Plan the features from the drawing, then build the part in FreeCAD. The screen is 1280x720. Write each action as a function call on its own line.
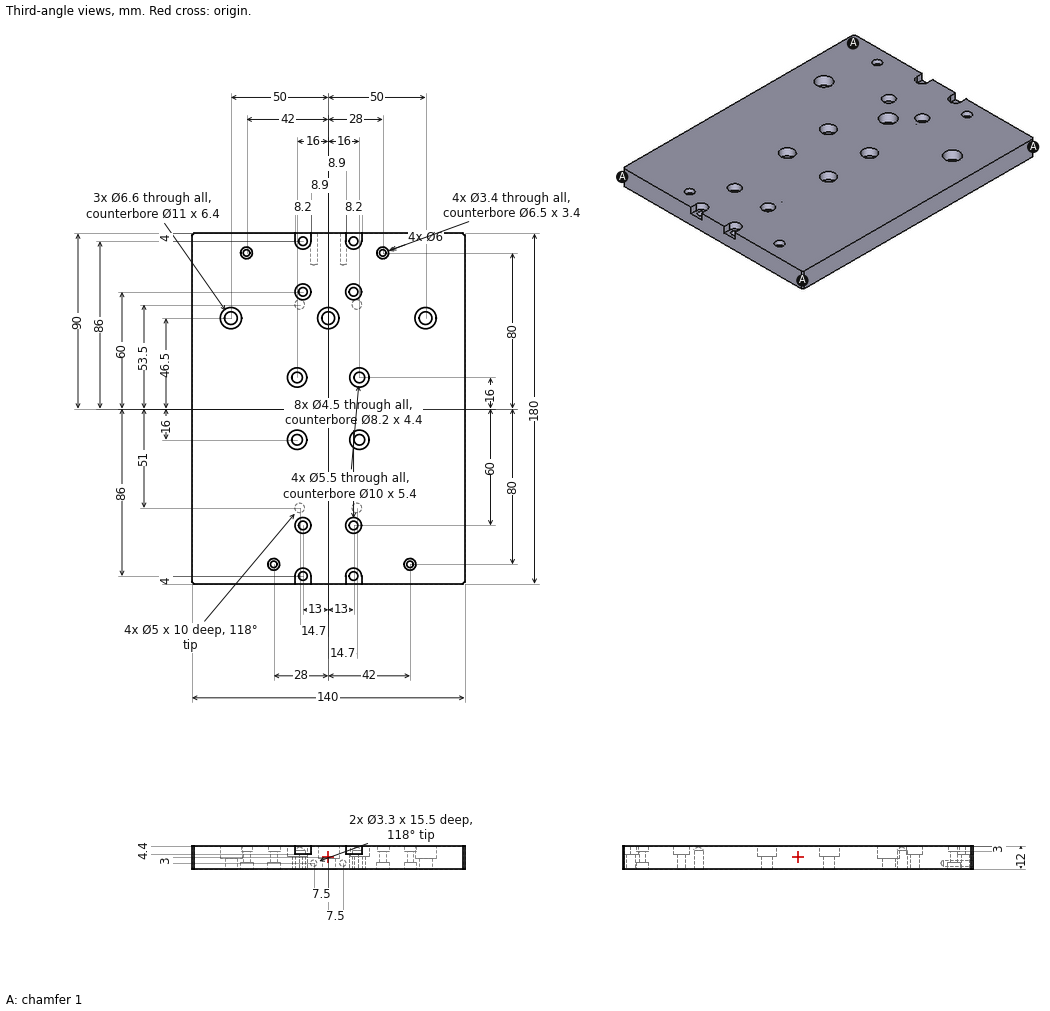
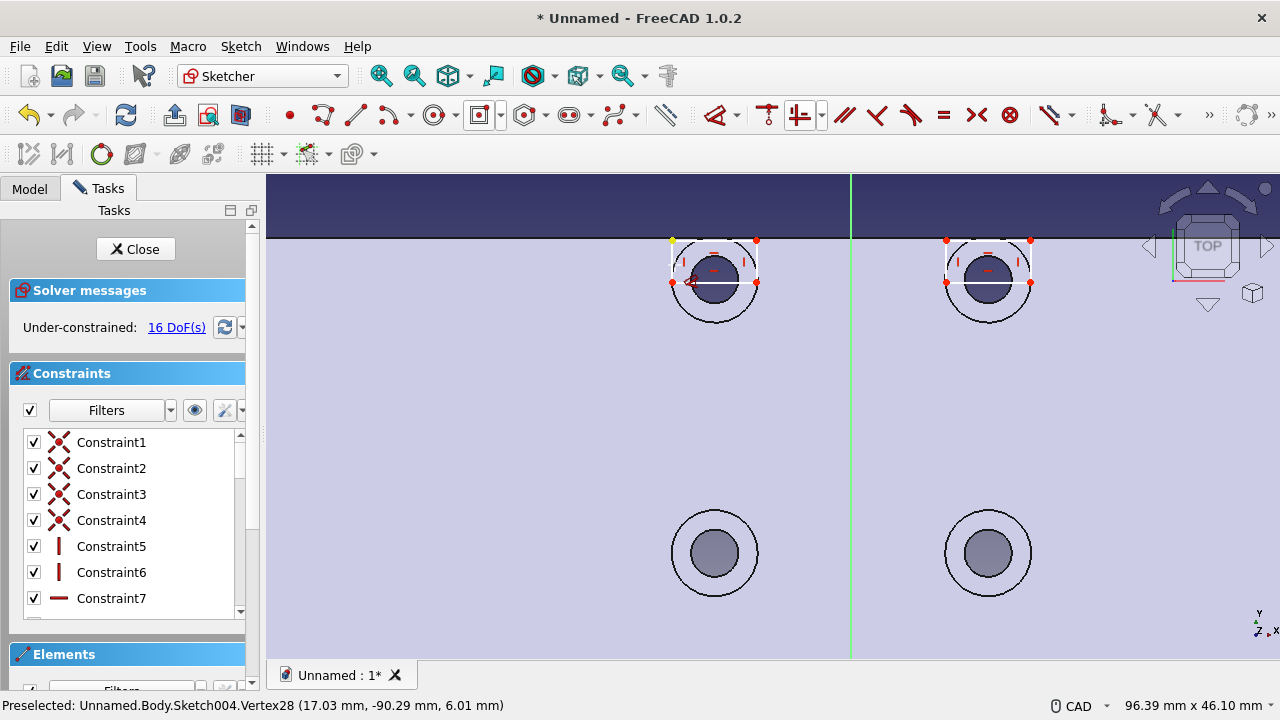
click(672, 262)
click(638, 262)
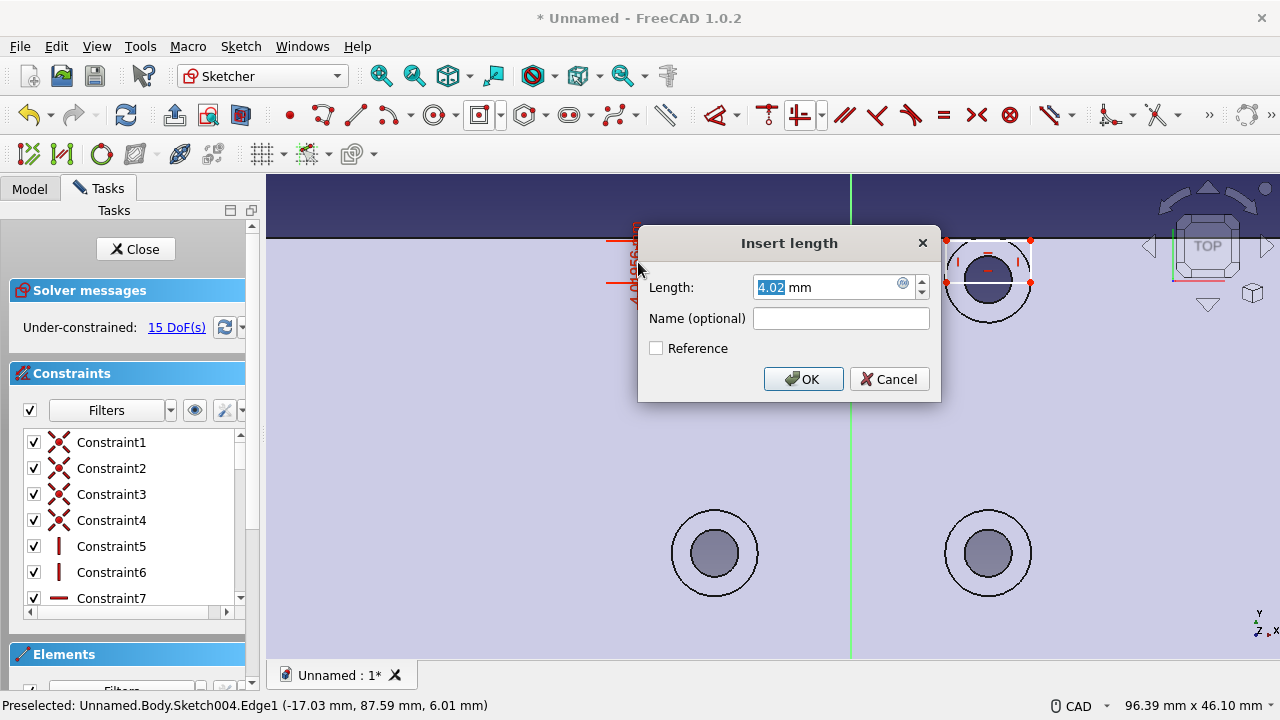
text(4)
key(Return)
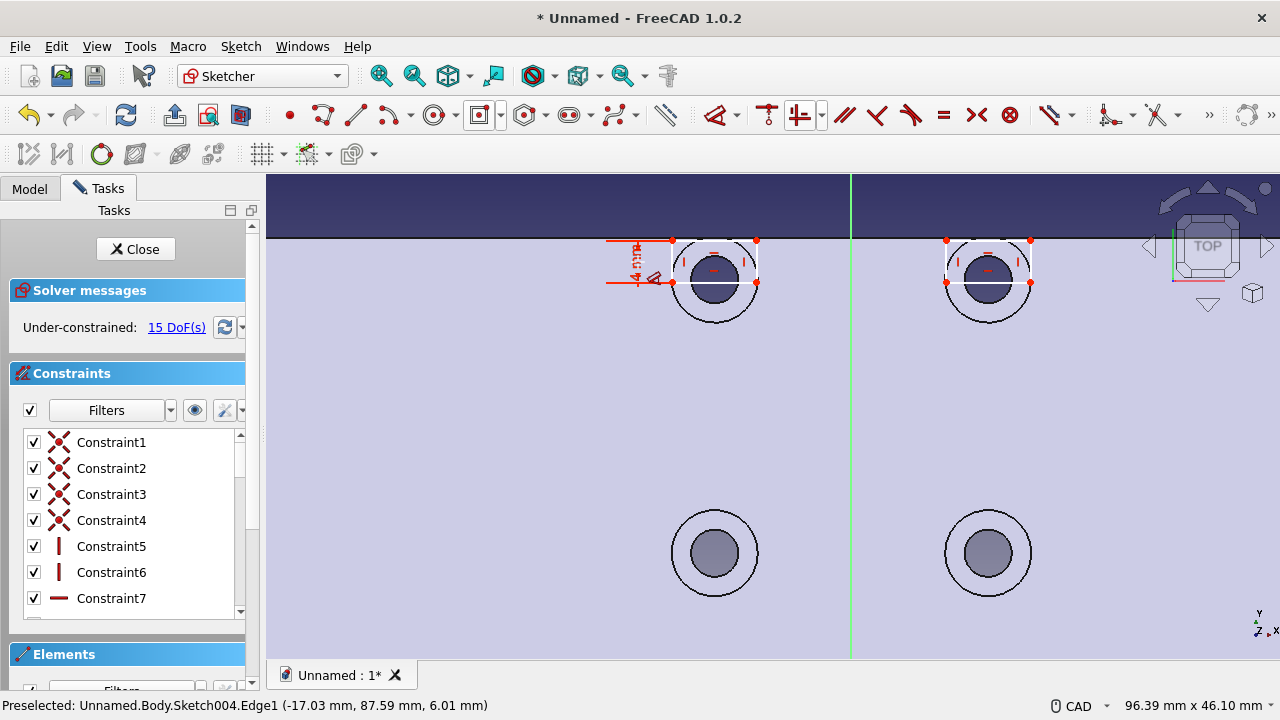
click(946, 253)
click(980, 262)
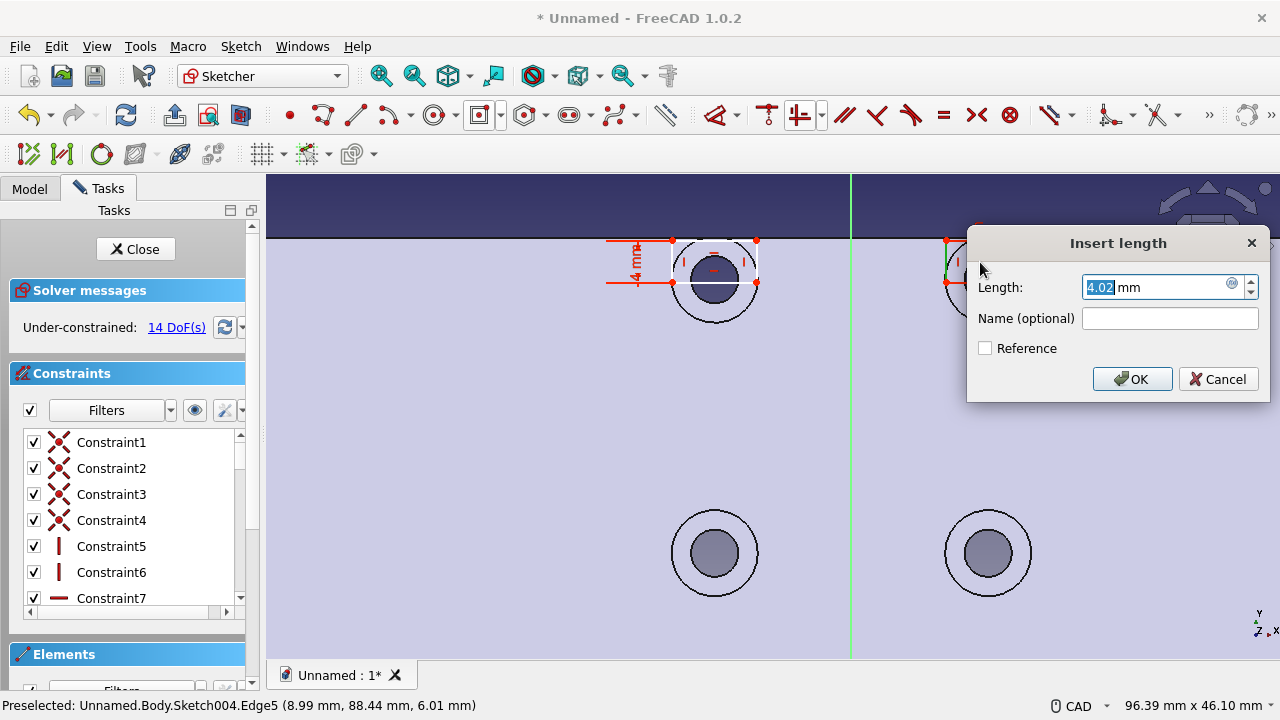
text(4)
key(Return)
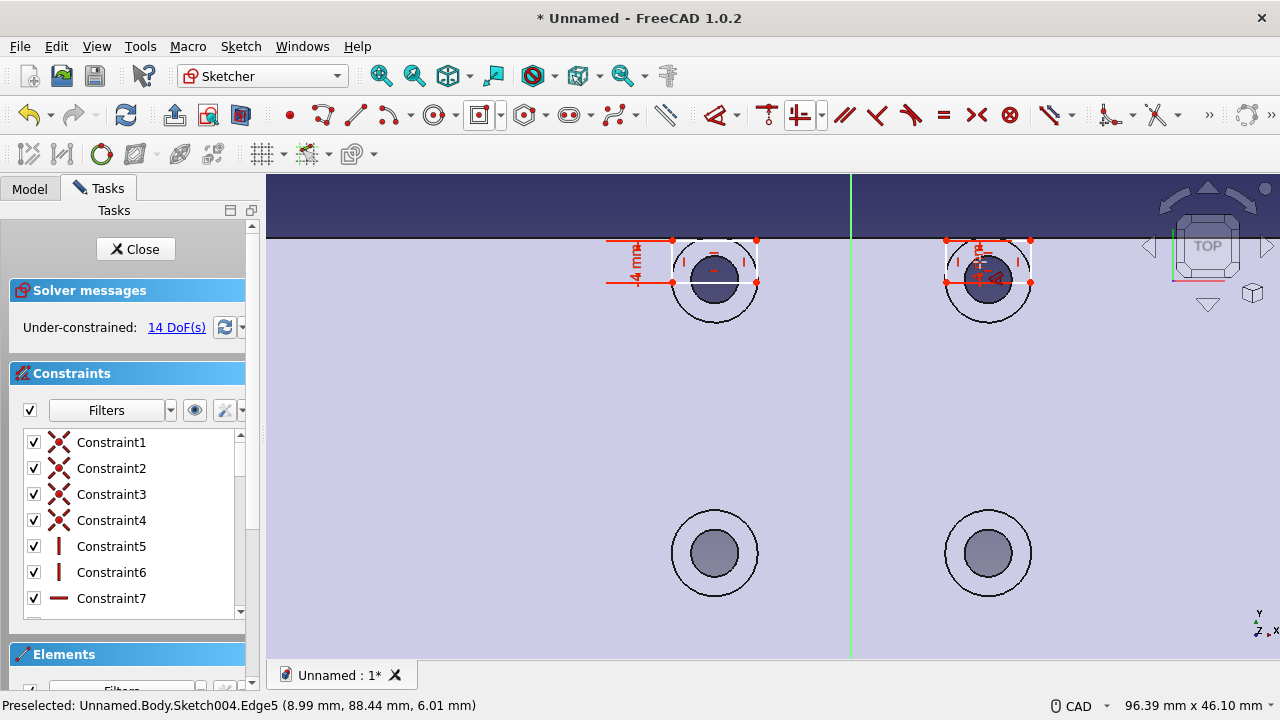
scroll(675, 264, down, 9)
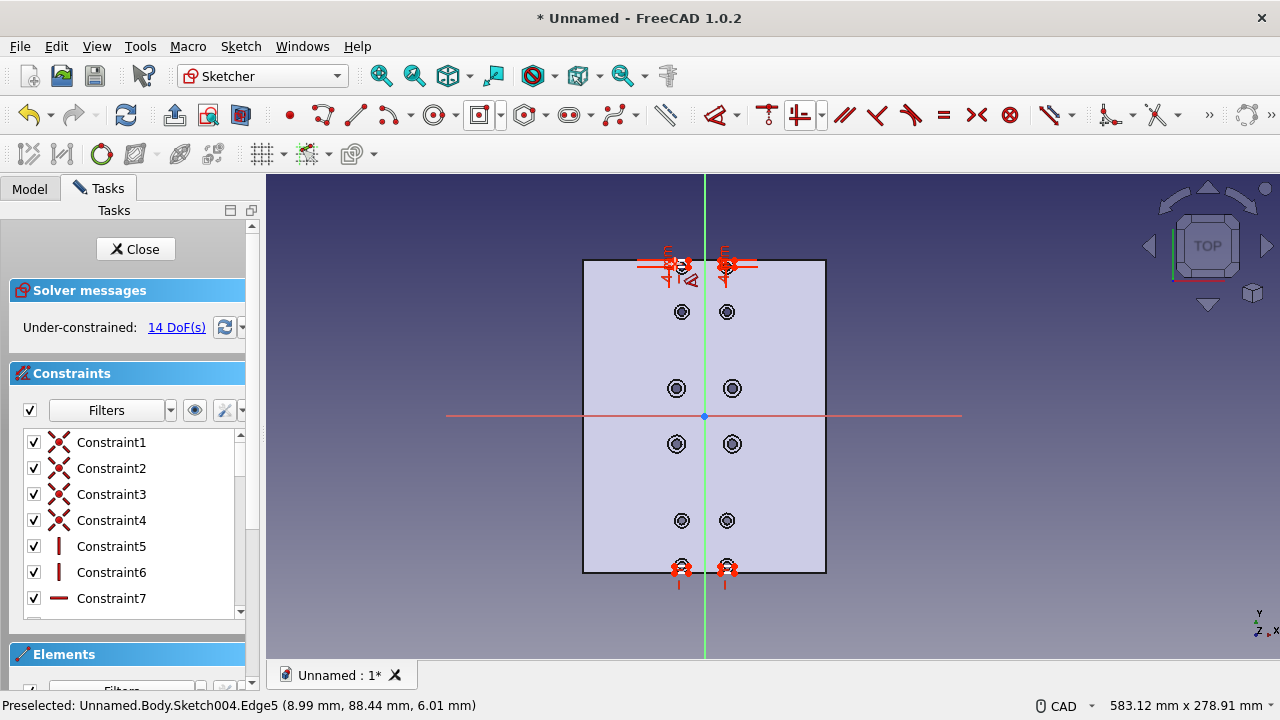
scroll(675, 568, up, 10)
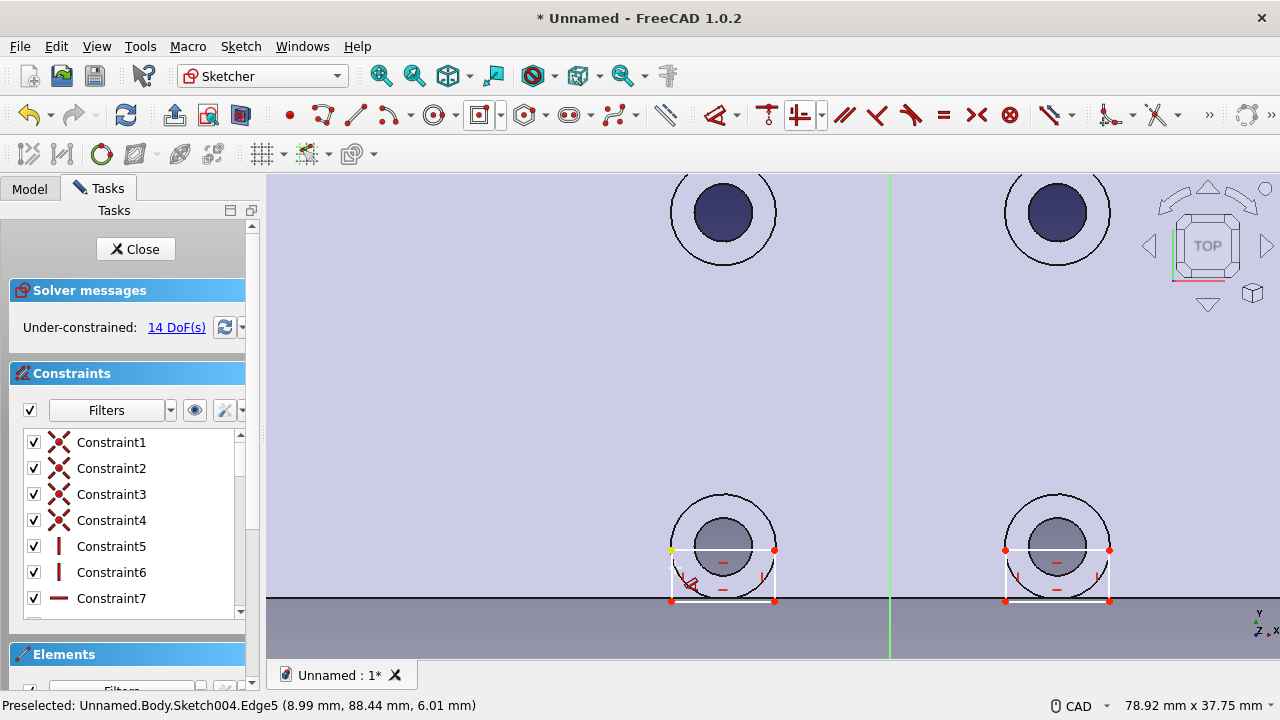
click(672, 566)
click(638, 576)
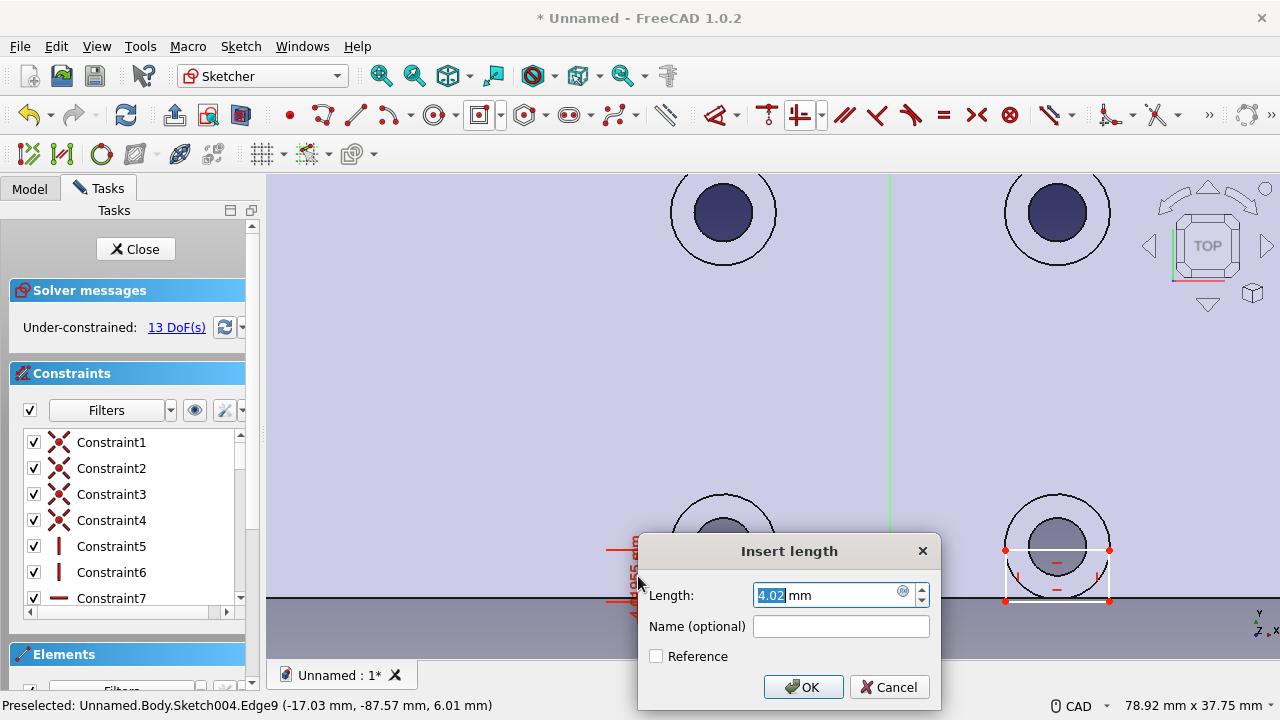
text(4)
key(Return)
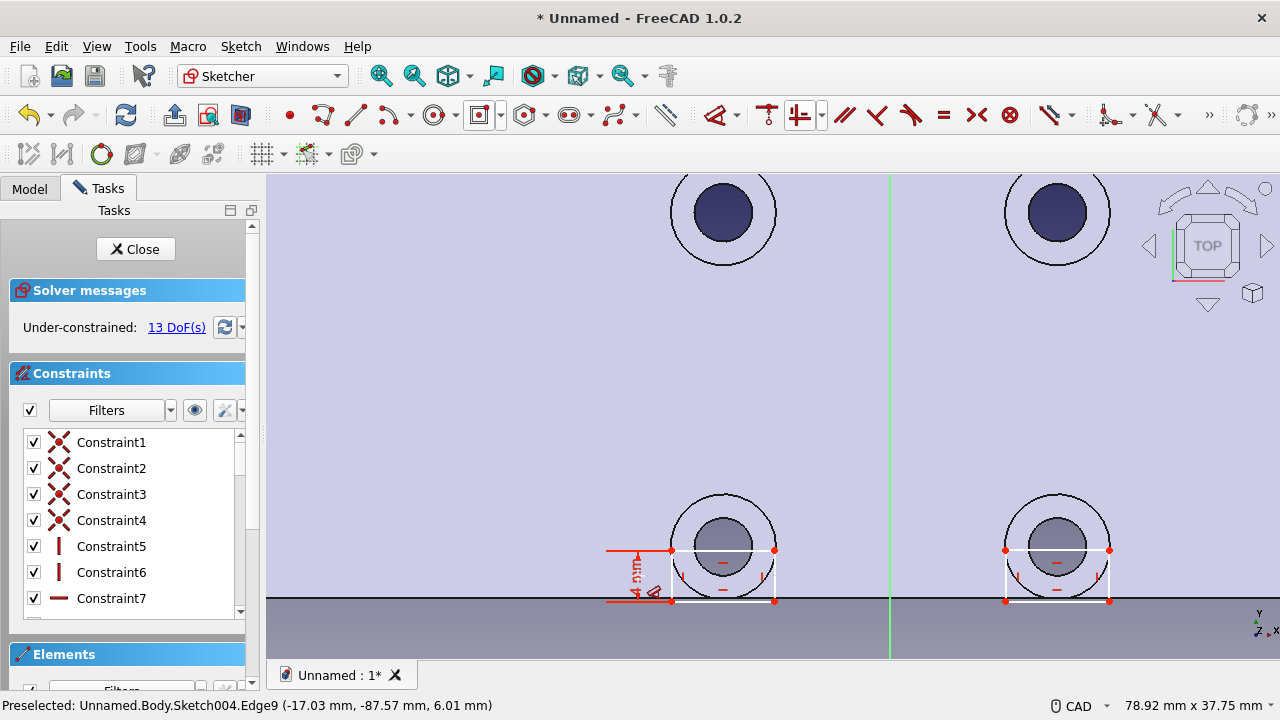
click(1006, 566)
click(1040, 576)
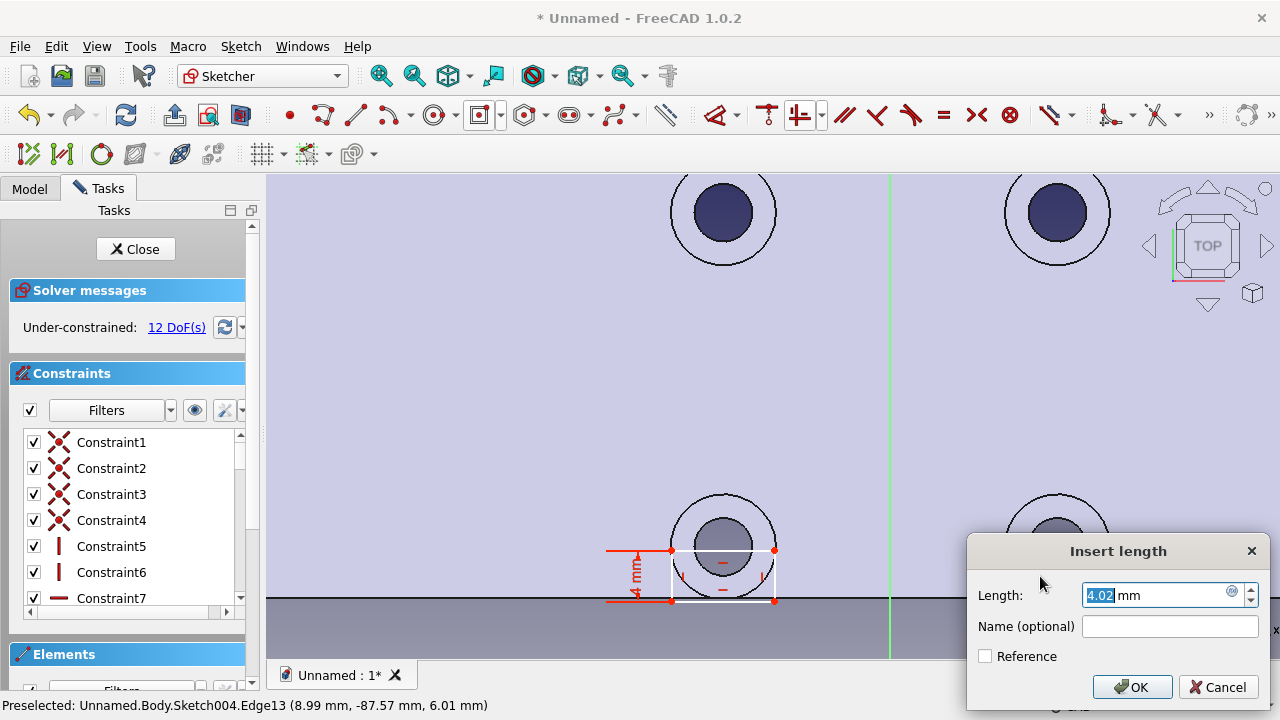
text(4)
key(Return)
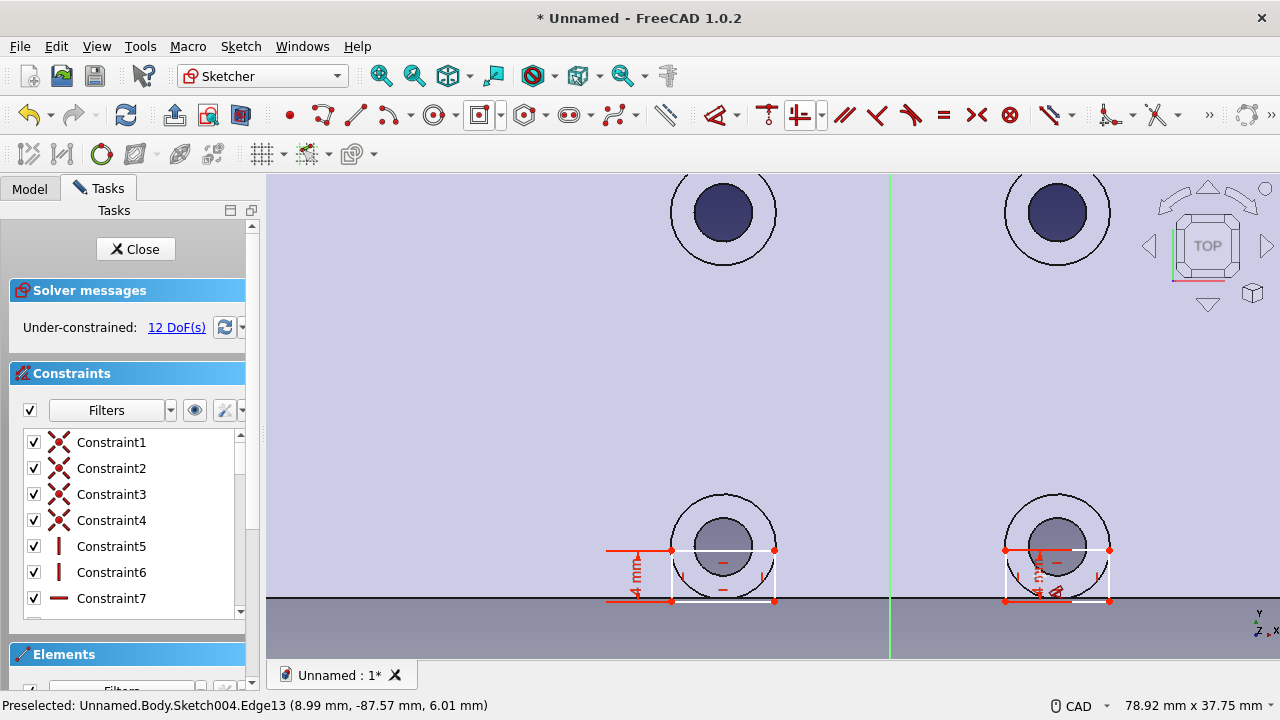
scroll(675, 569, down, 10)